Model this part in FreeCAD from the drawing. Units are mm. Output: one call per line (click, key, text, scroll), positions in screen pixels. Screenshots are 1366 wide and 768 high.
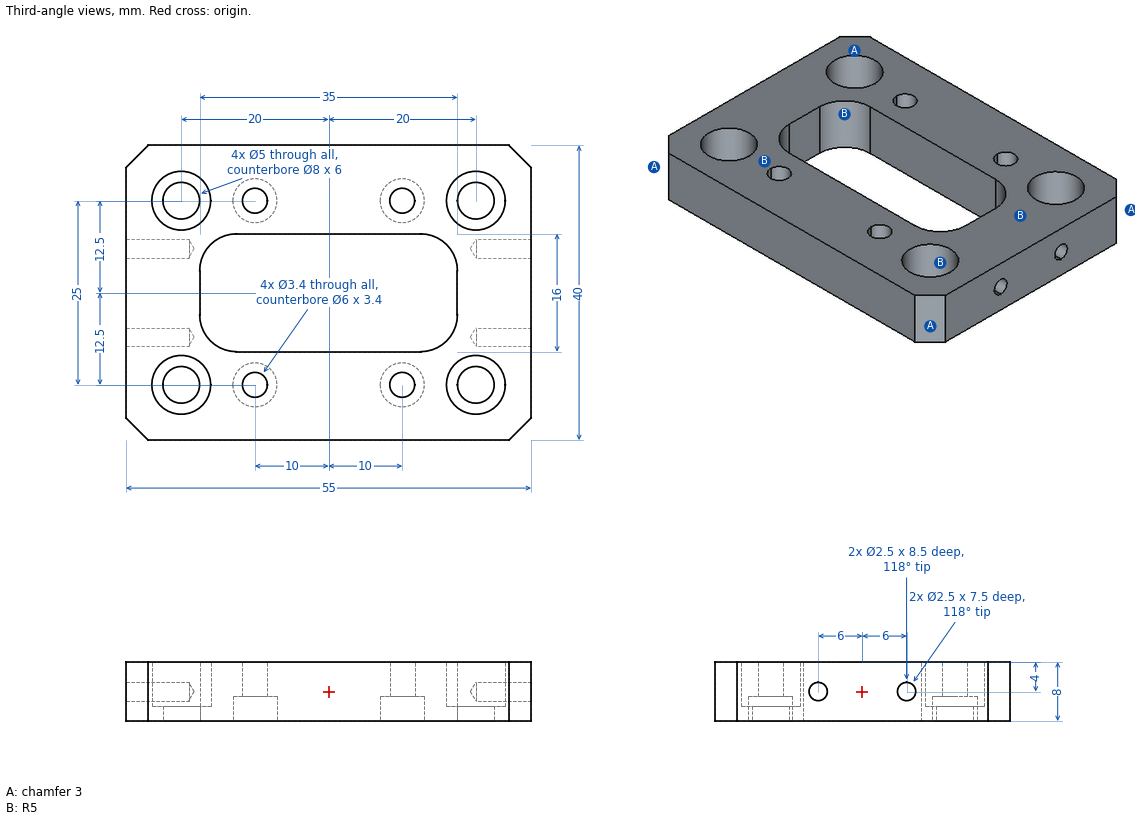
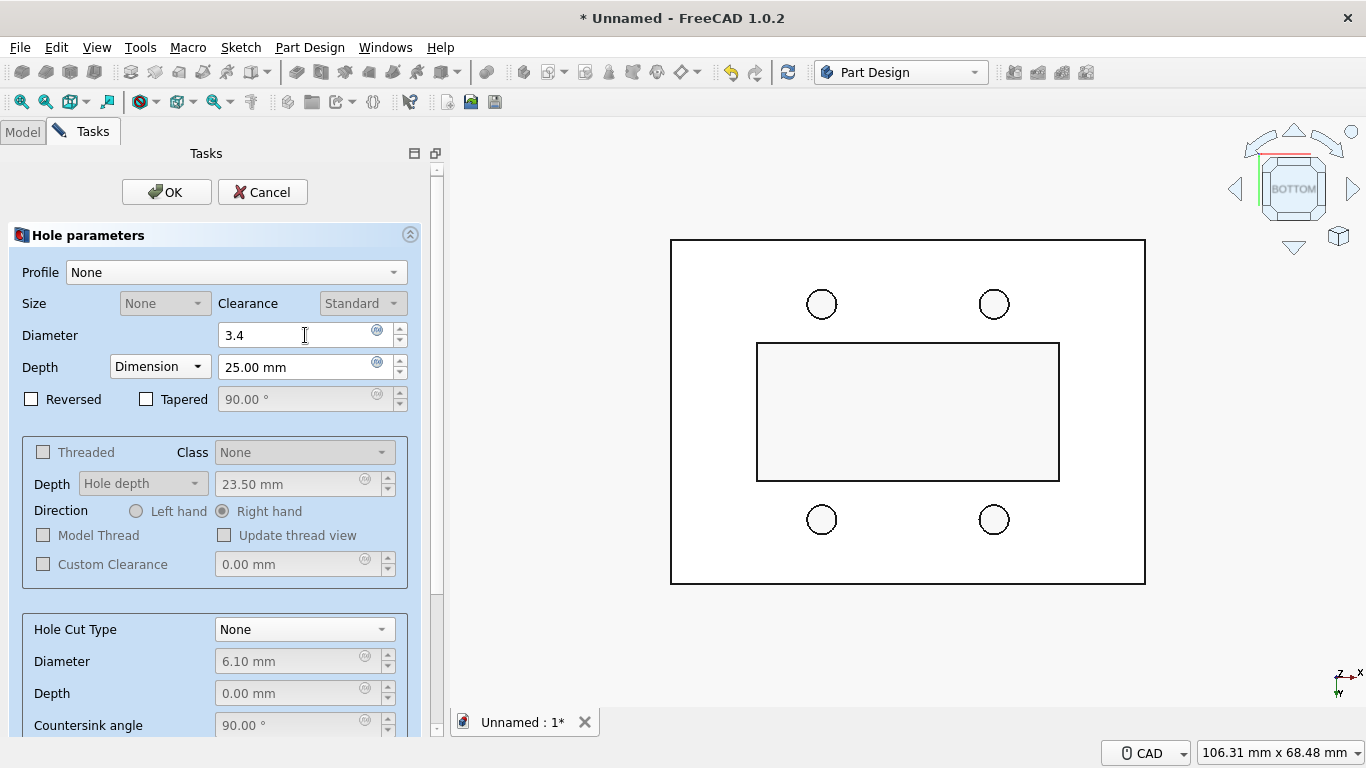
click(161, 366)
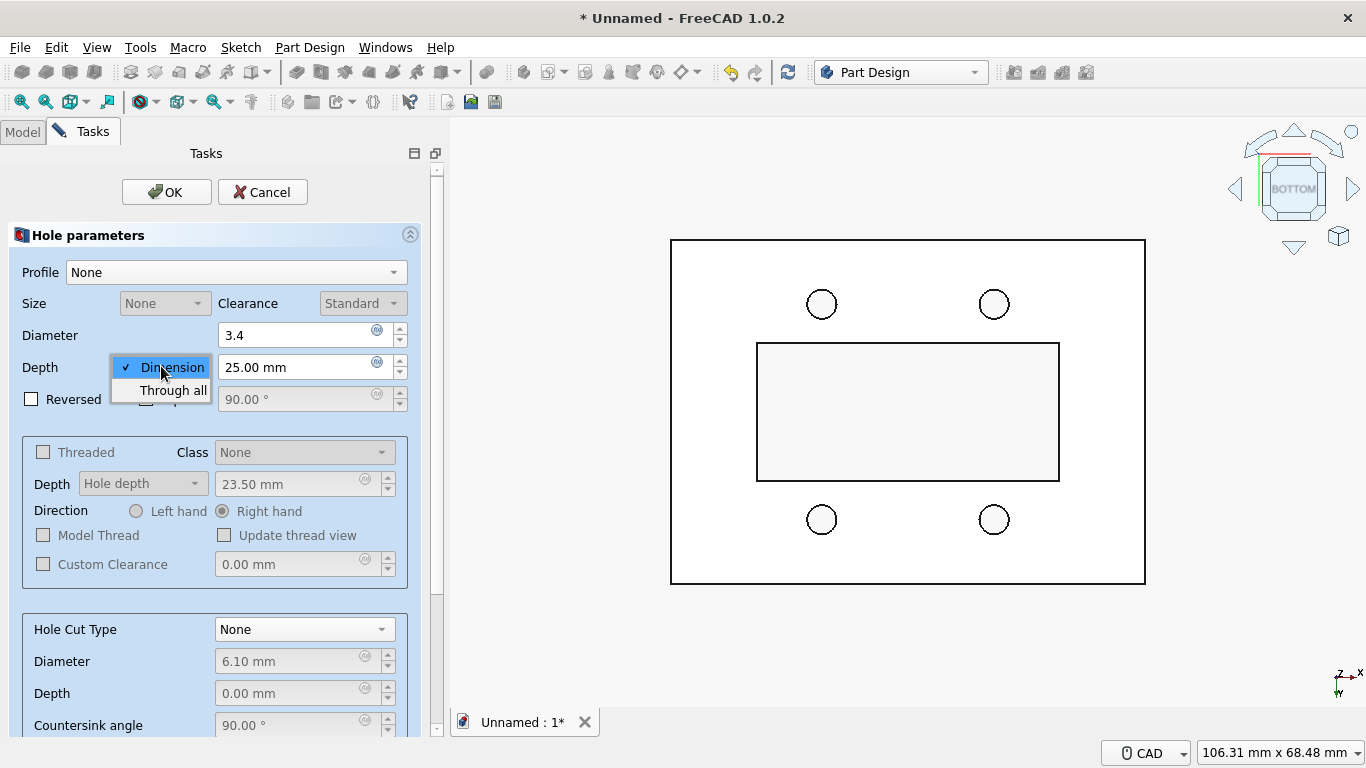
click(160, 390)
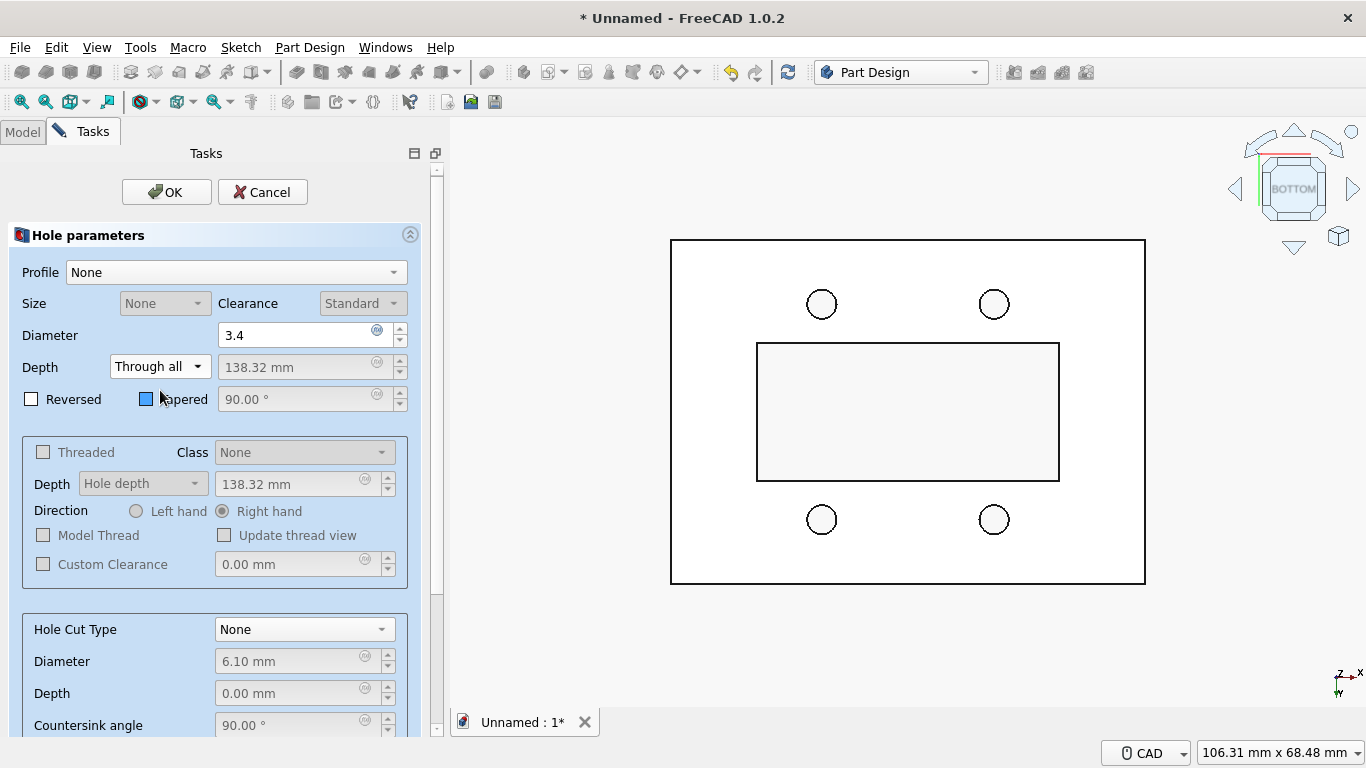
click(306, 630)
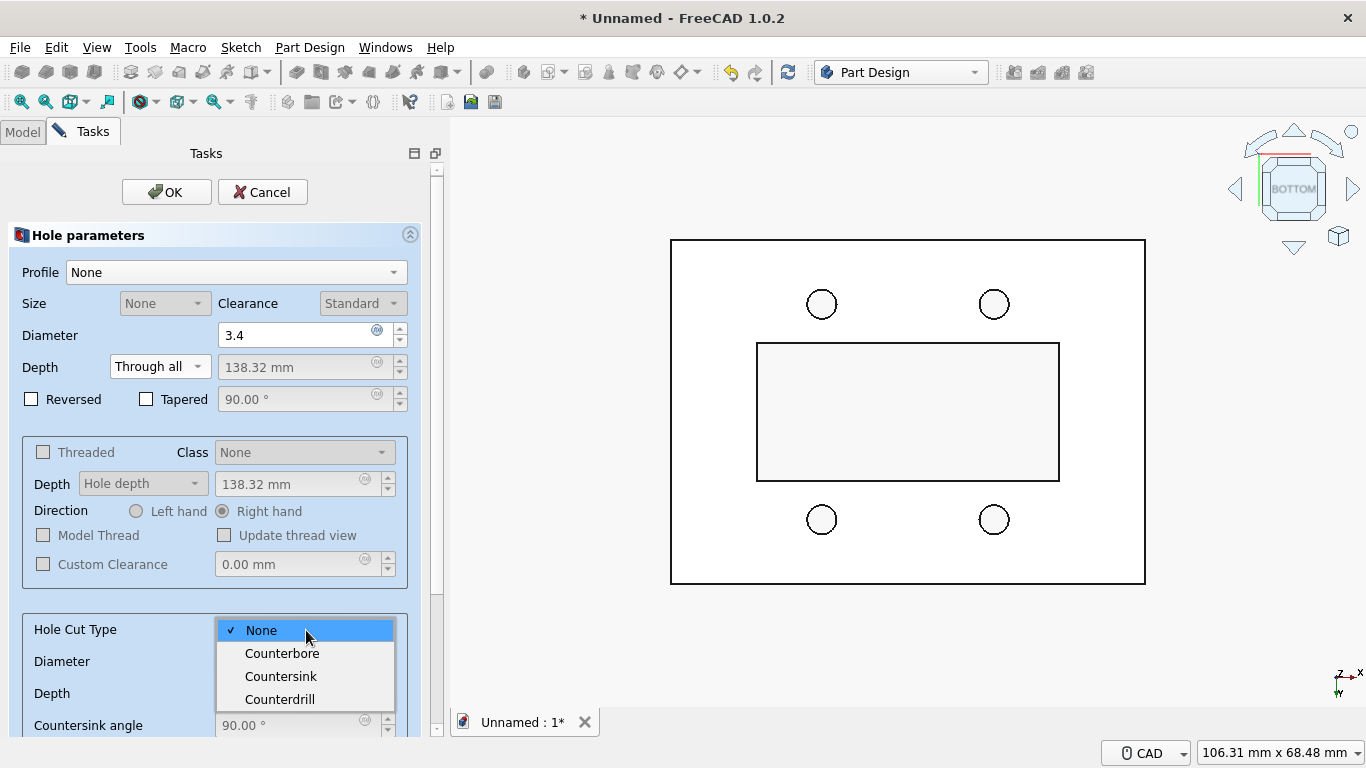
click(304, 654)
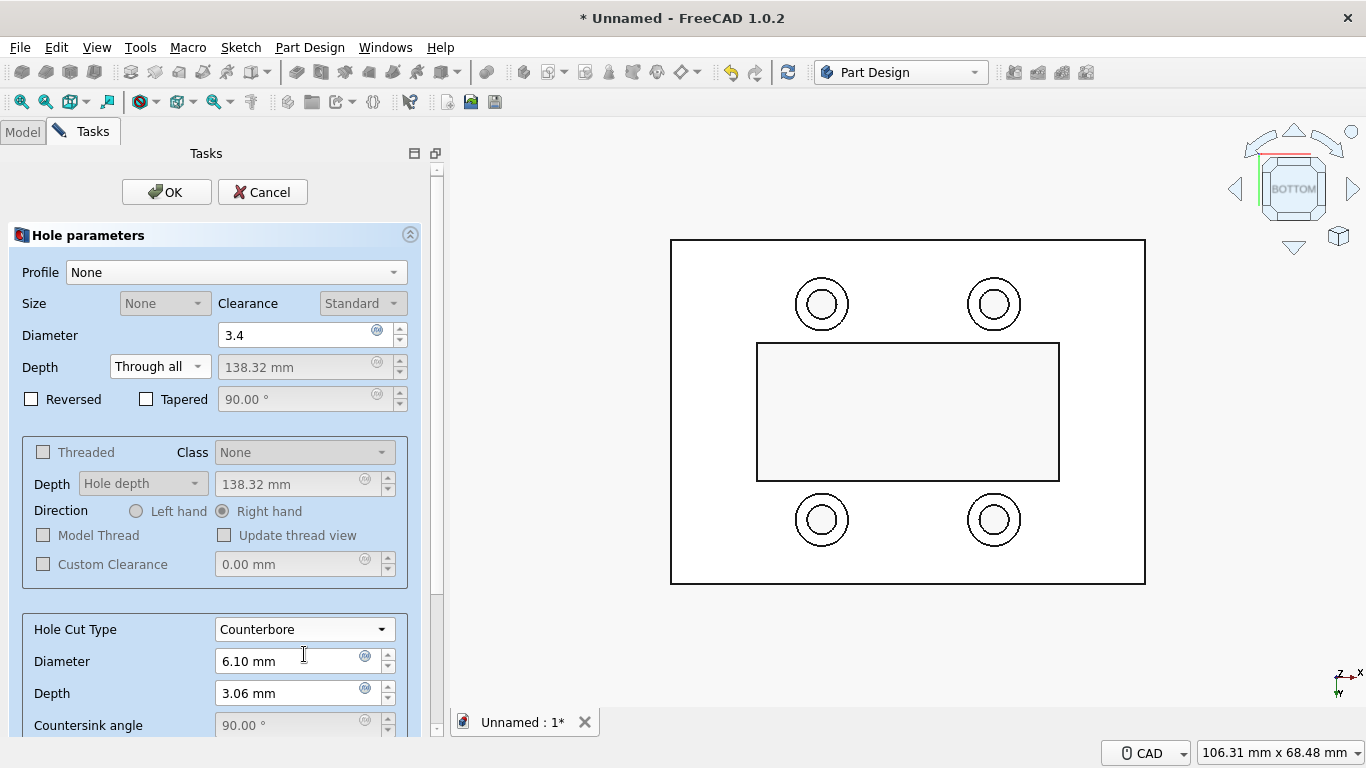
triple_click(298, 661)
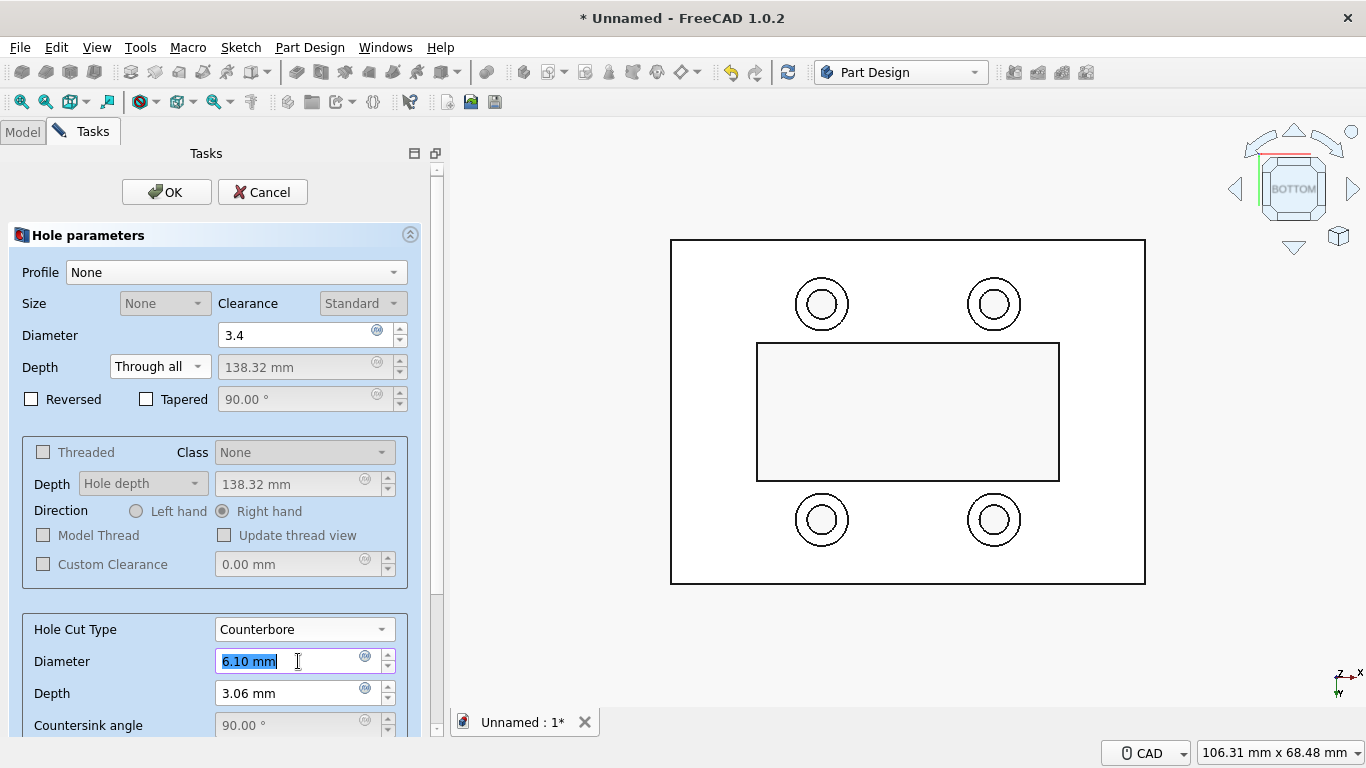
text(6)
key(Tab)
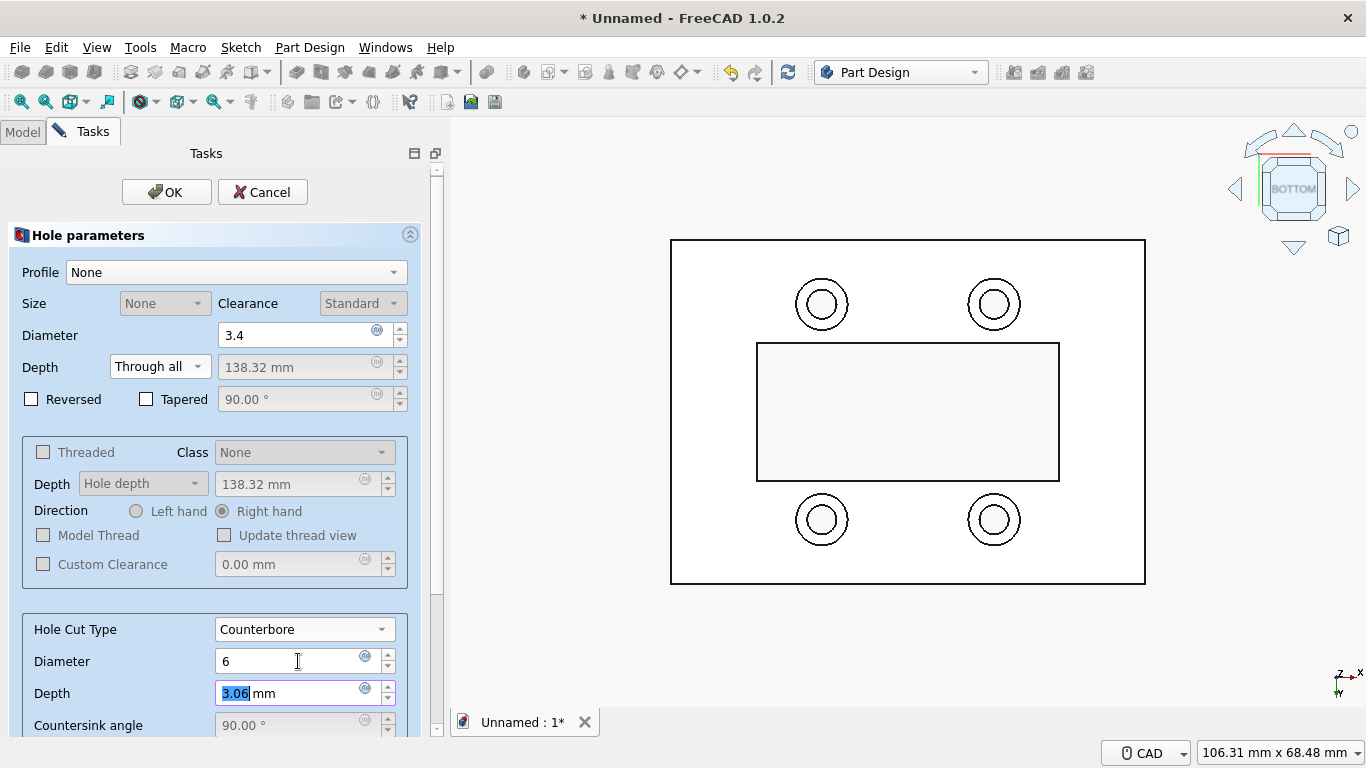
text(3.4)
key(Tab)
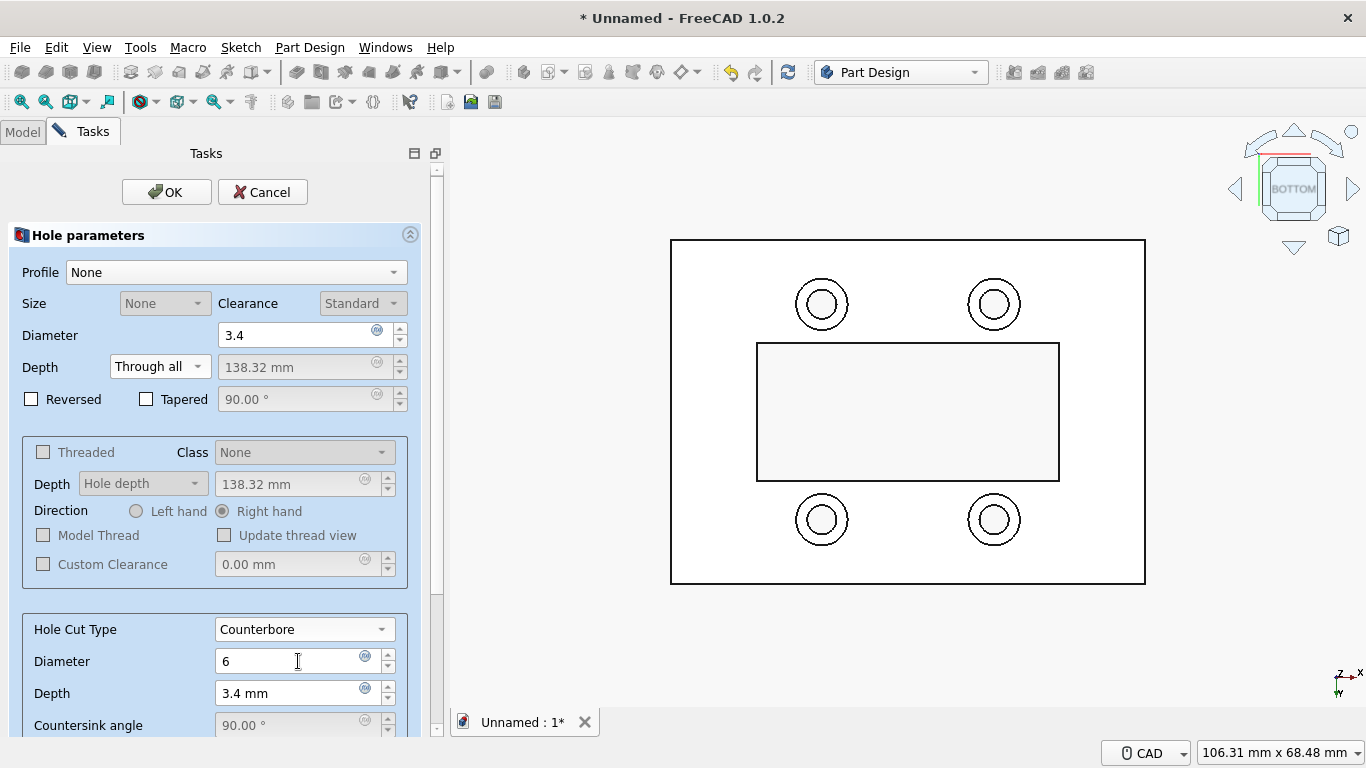
click(167, 192)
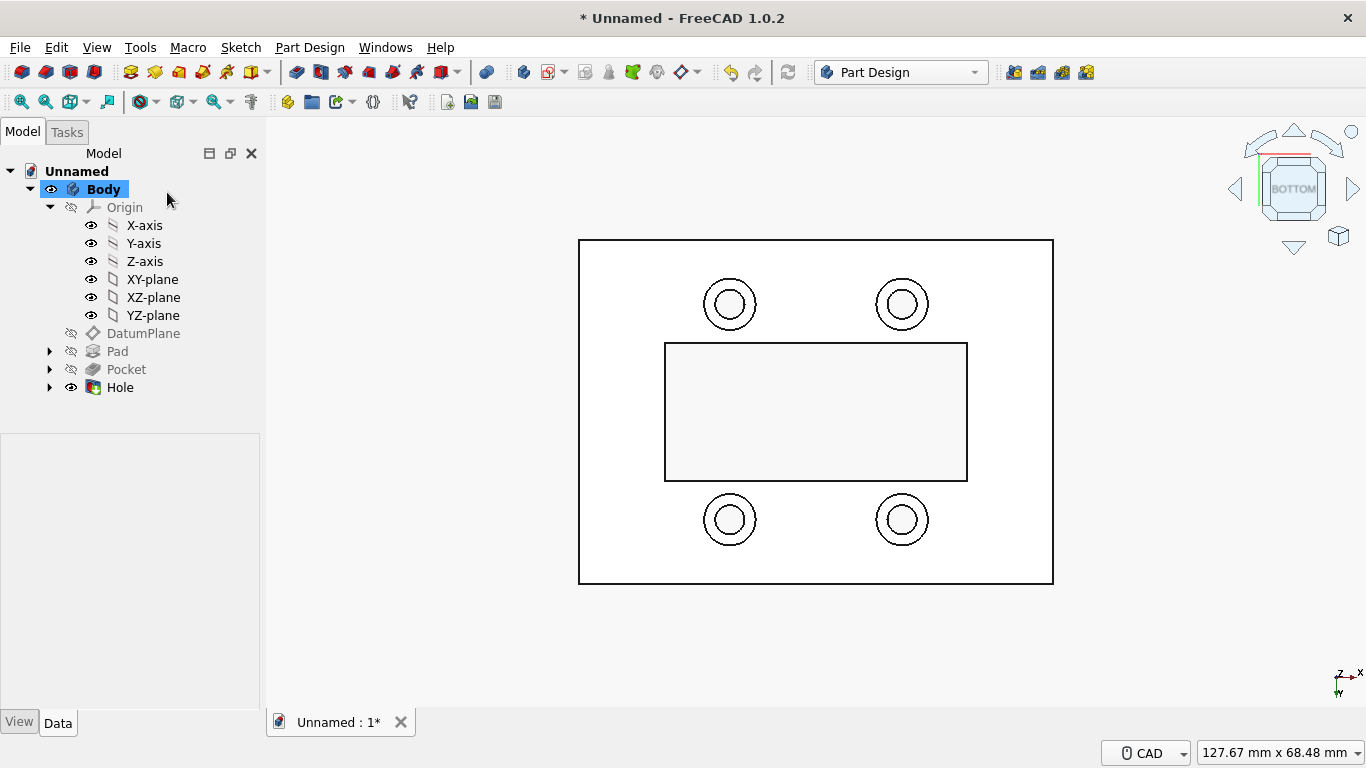
key(0)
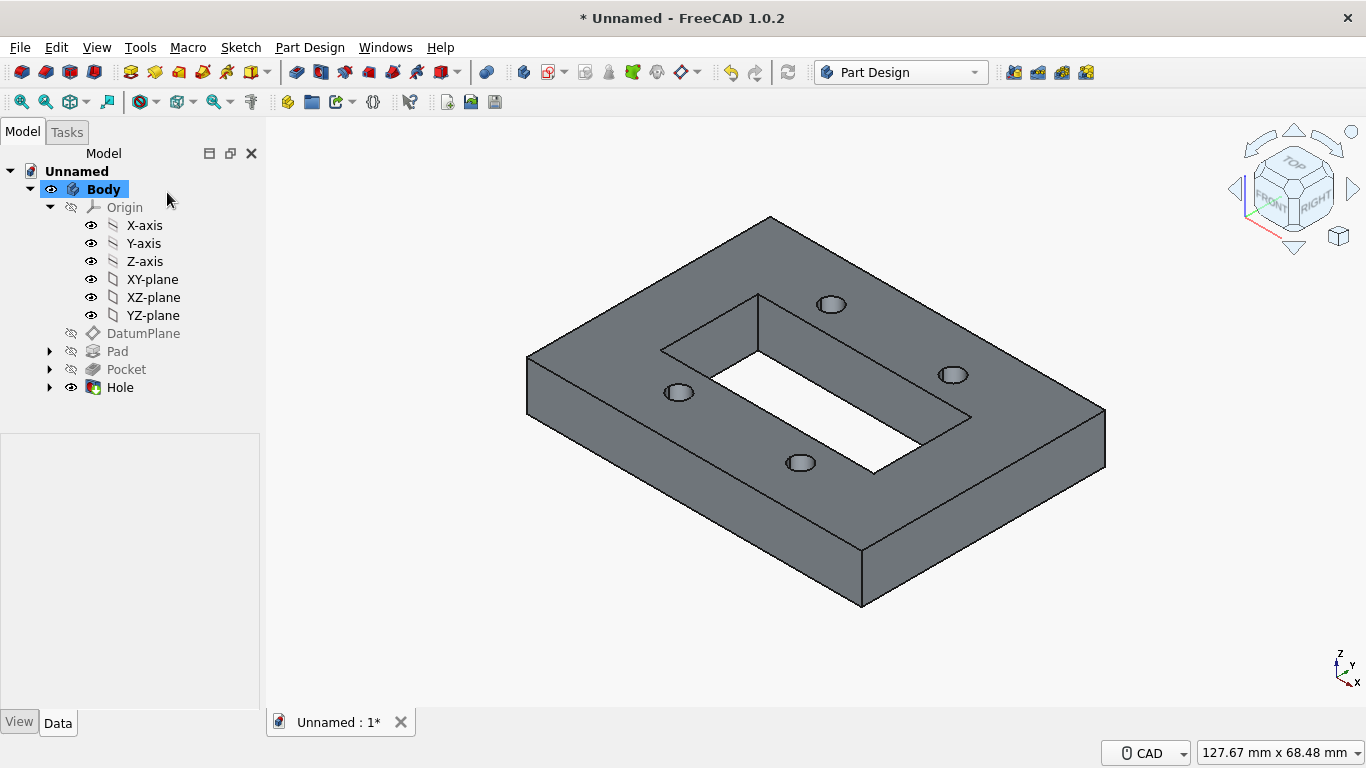
click(1053, 468)